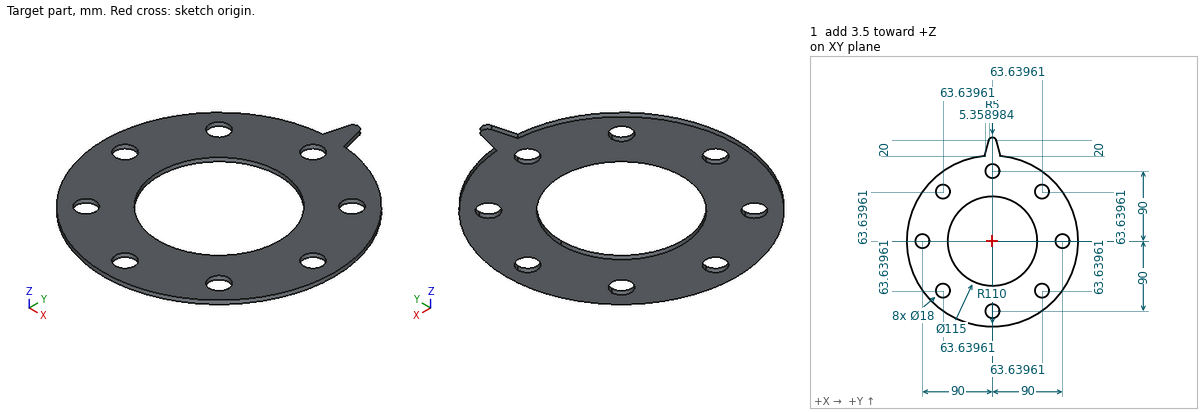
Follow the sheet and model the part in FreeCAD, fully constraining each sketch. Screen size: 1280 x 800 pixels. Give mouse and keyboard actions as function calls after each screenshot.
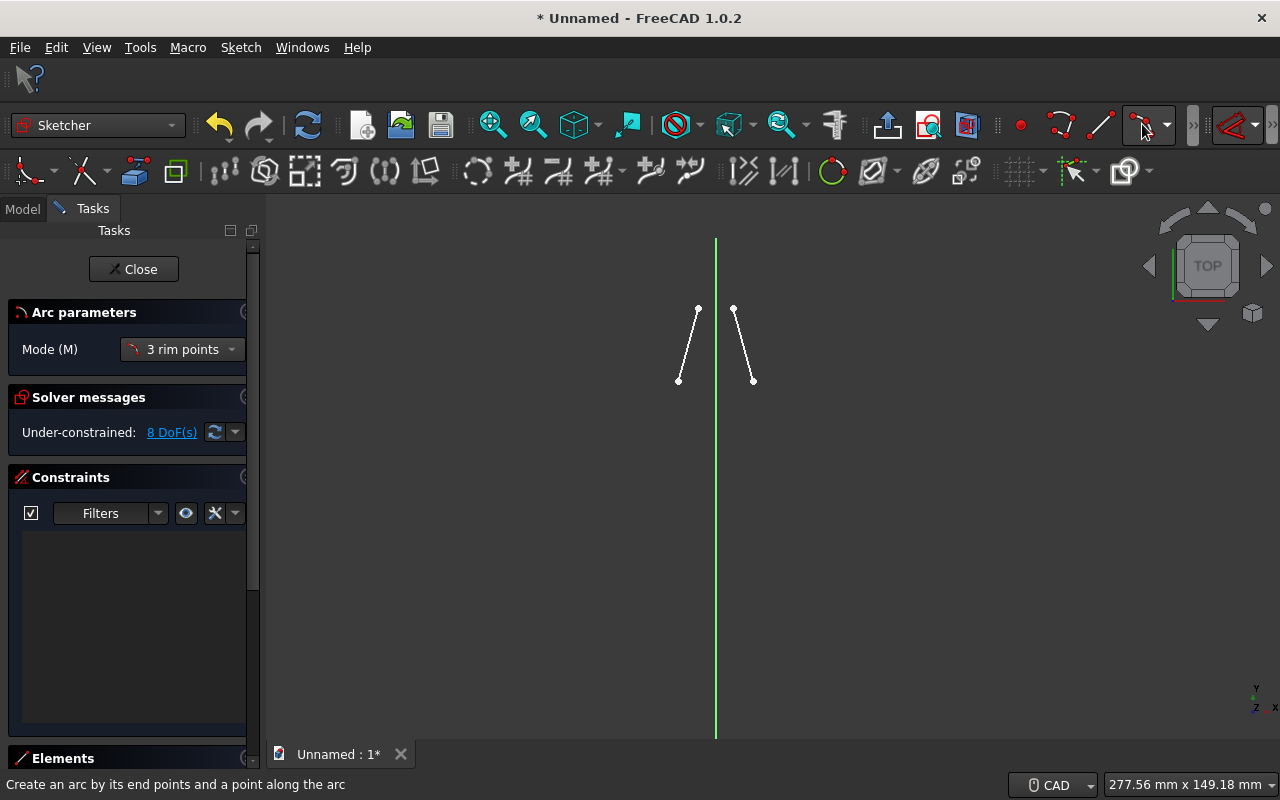
click(678, 381)
click(753, 381)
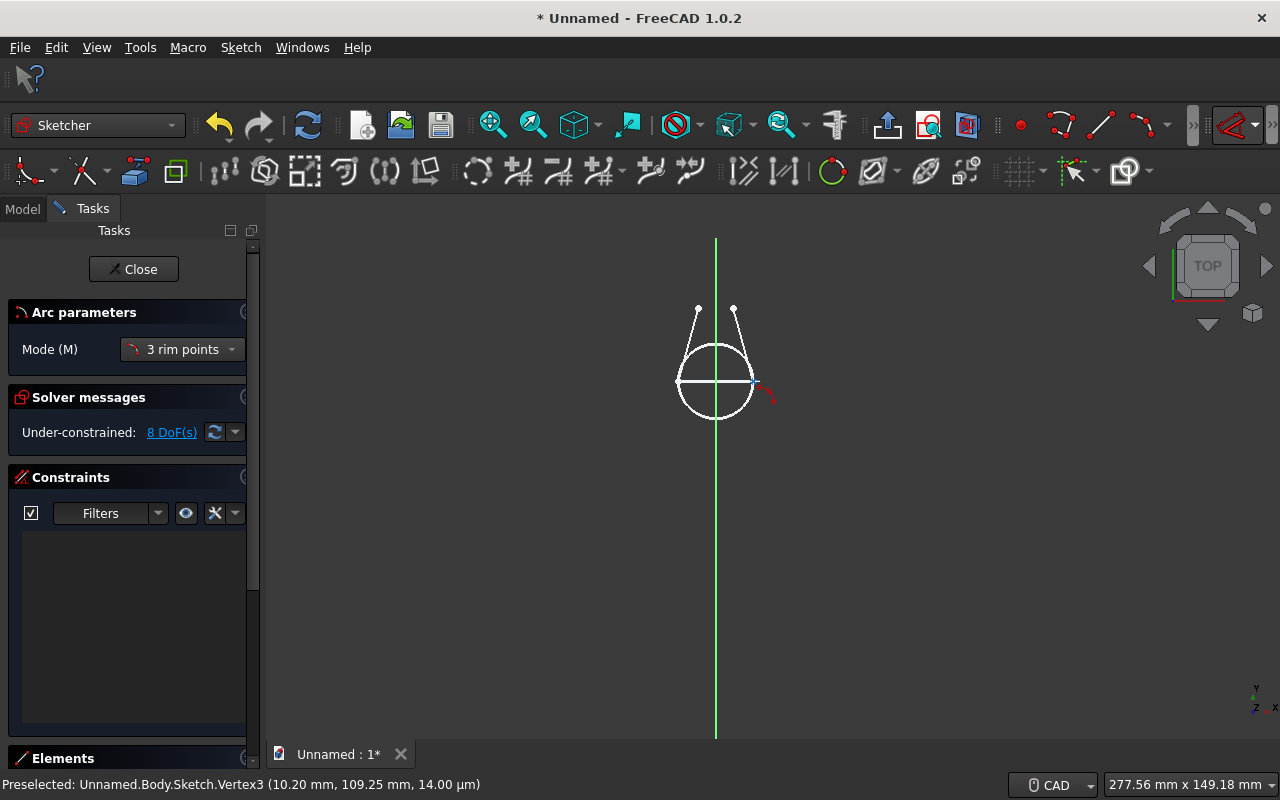
scroll(698, 309, down, 5)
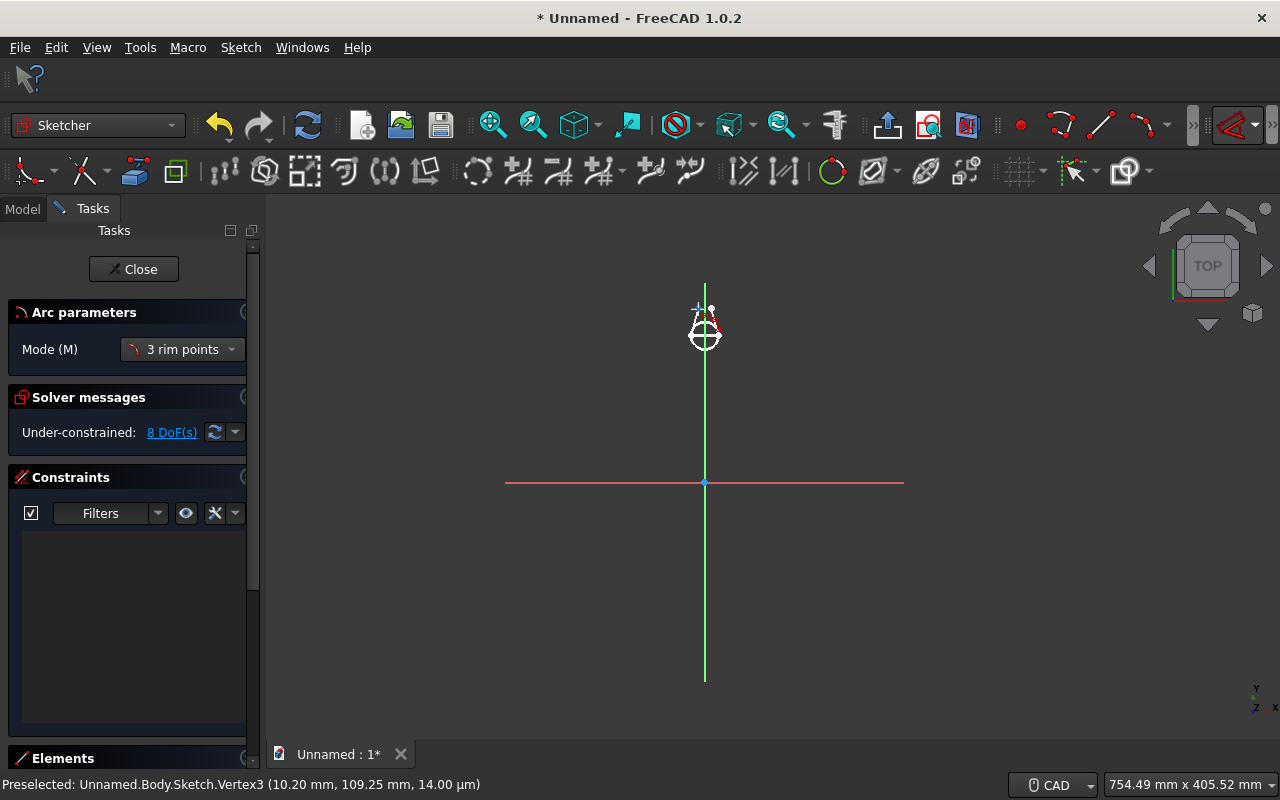
click(620, 604)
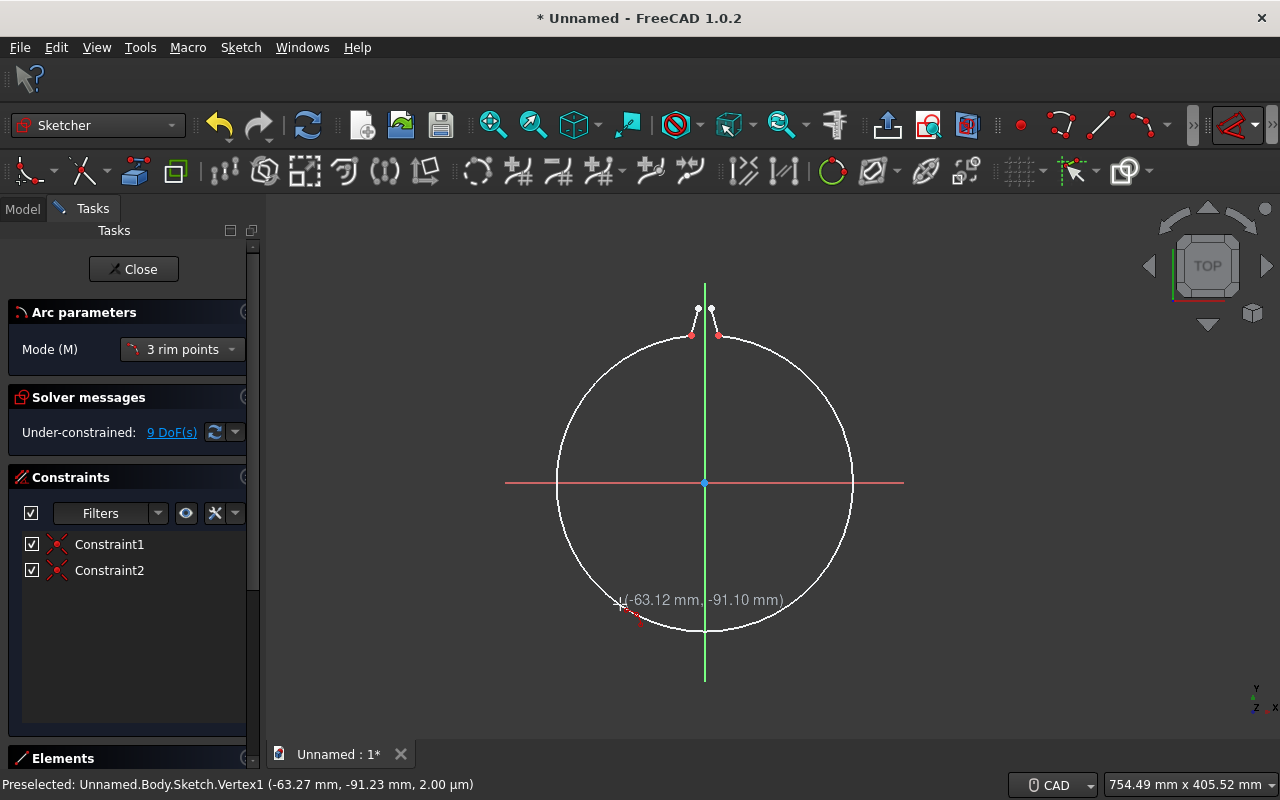
scroll(711, 308, up, 5)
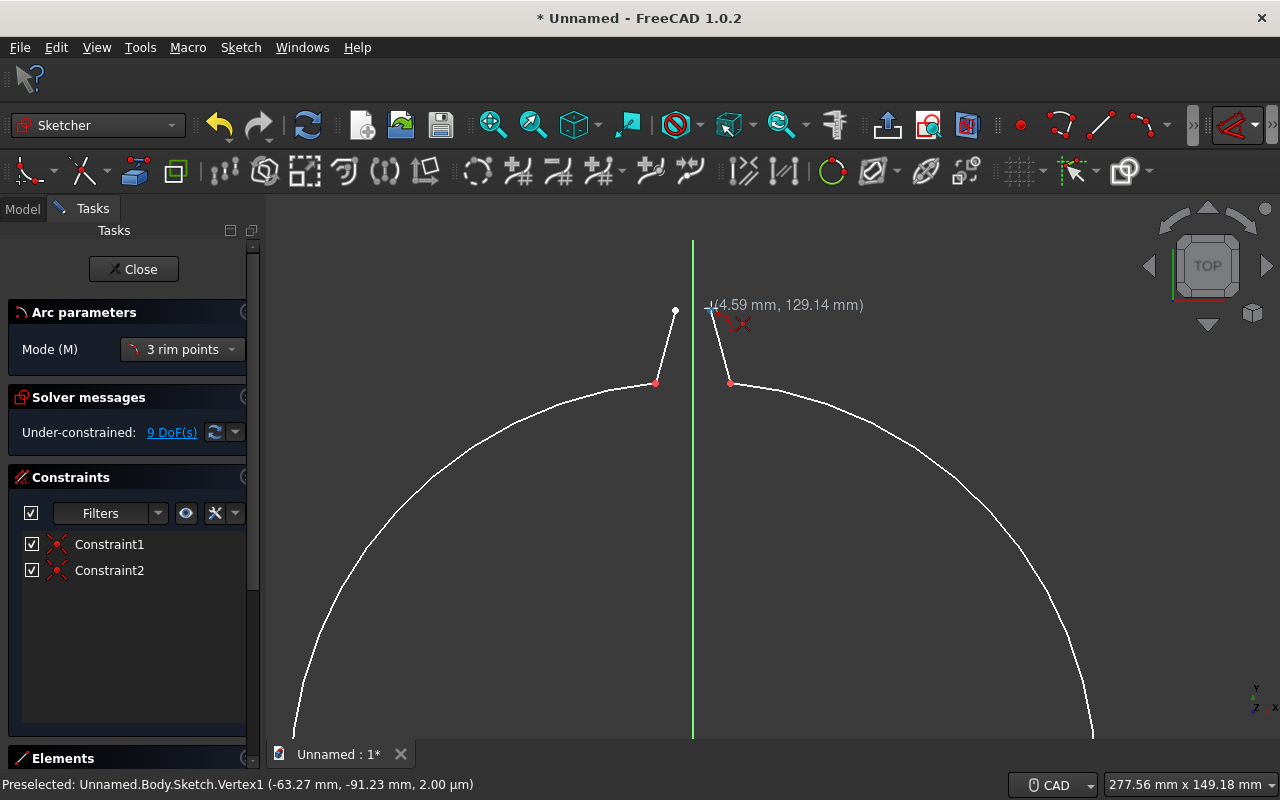
click(711, 310)
click(676, 310)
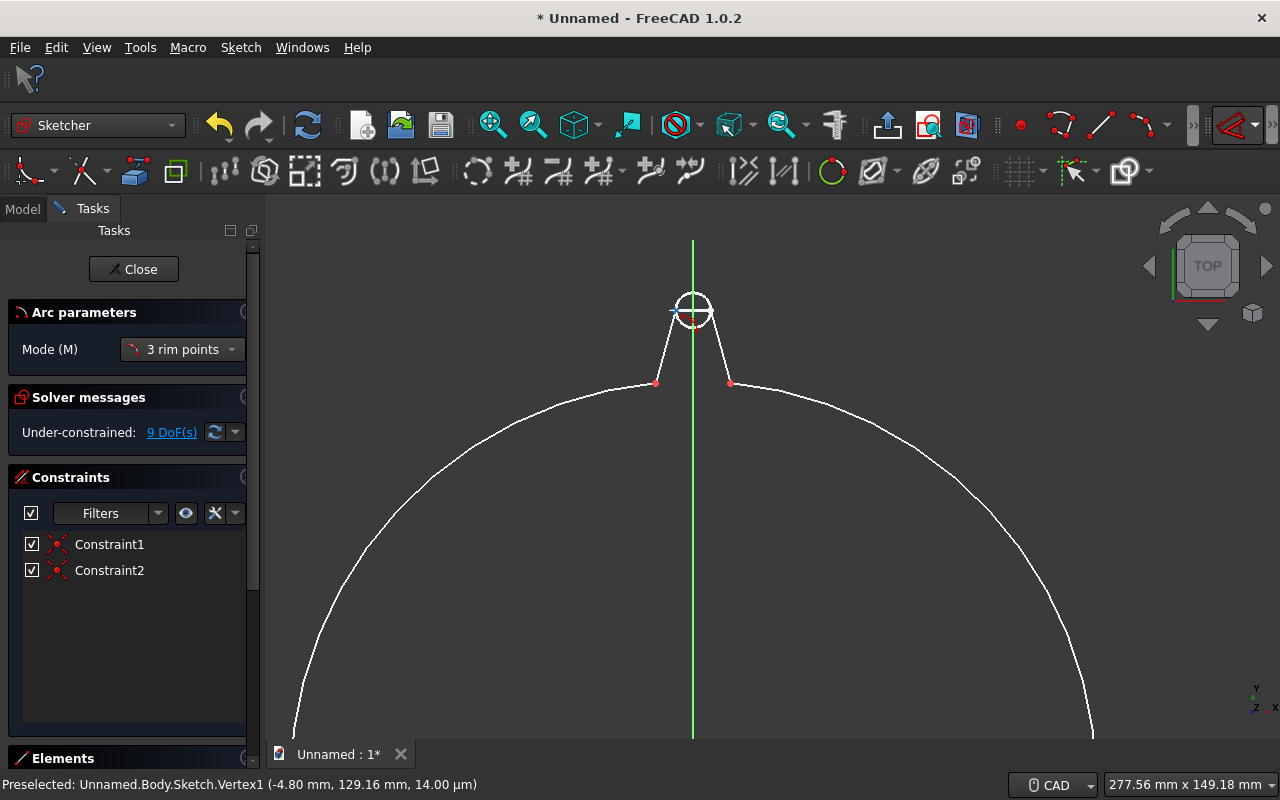
scroll(703, 298, up, 3)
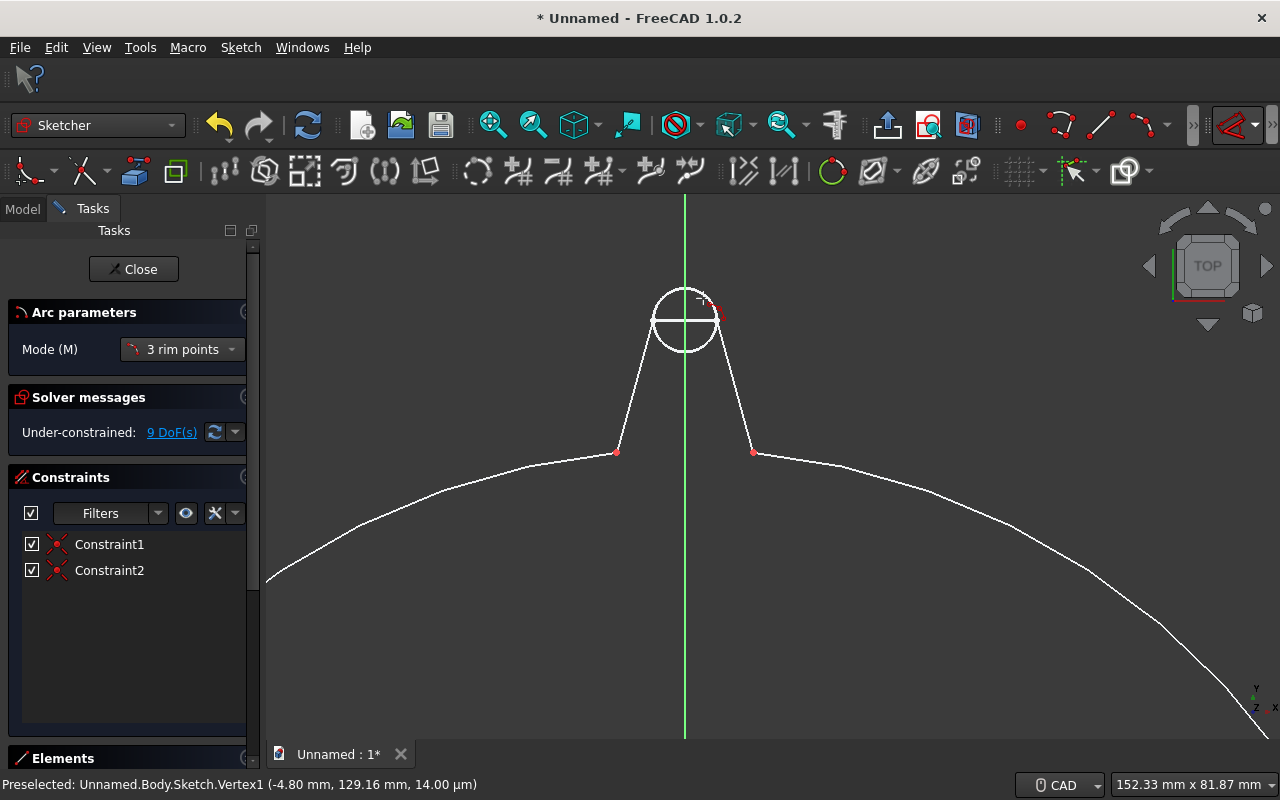
click(702, 298)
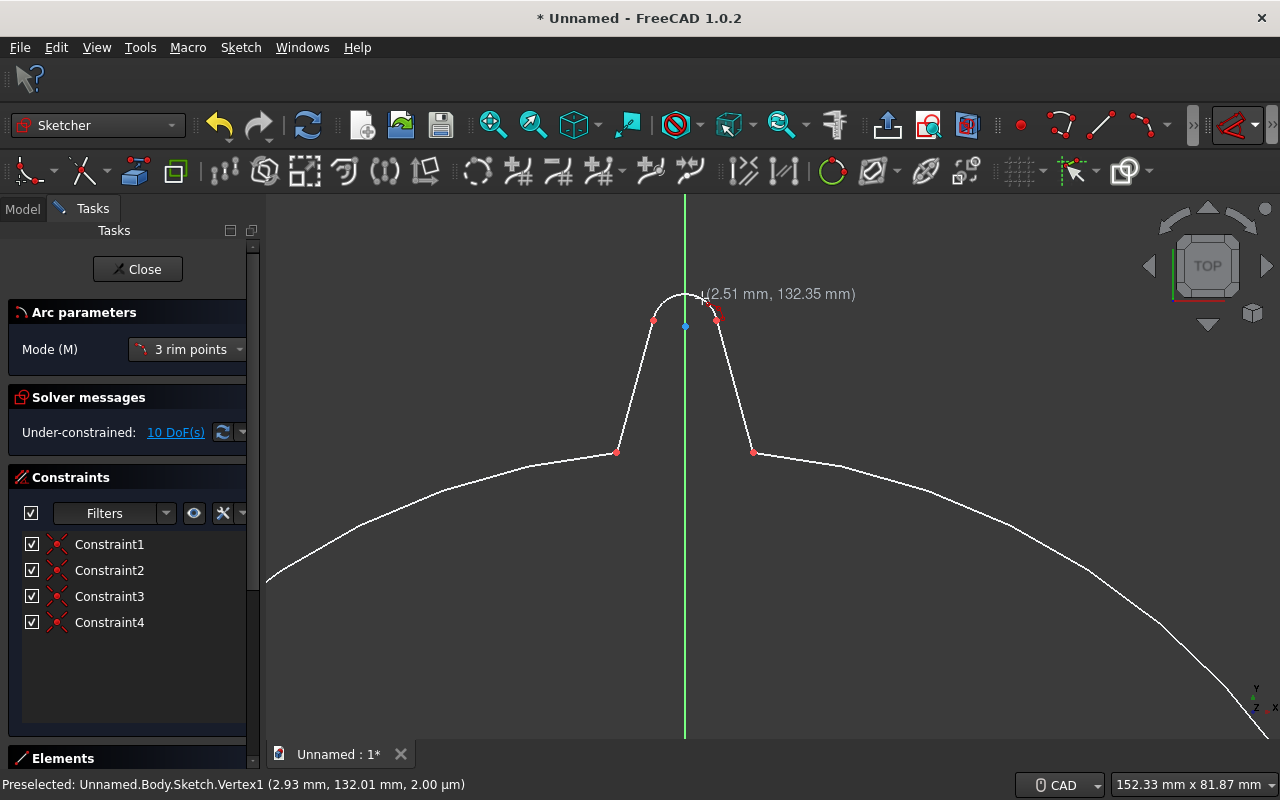
key(g)
key(c)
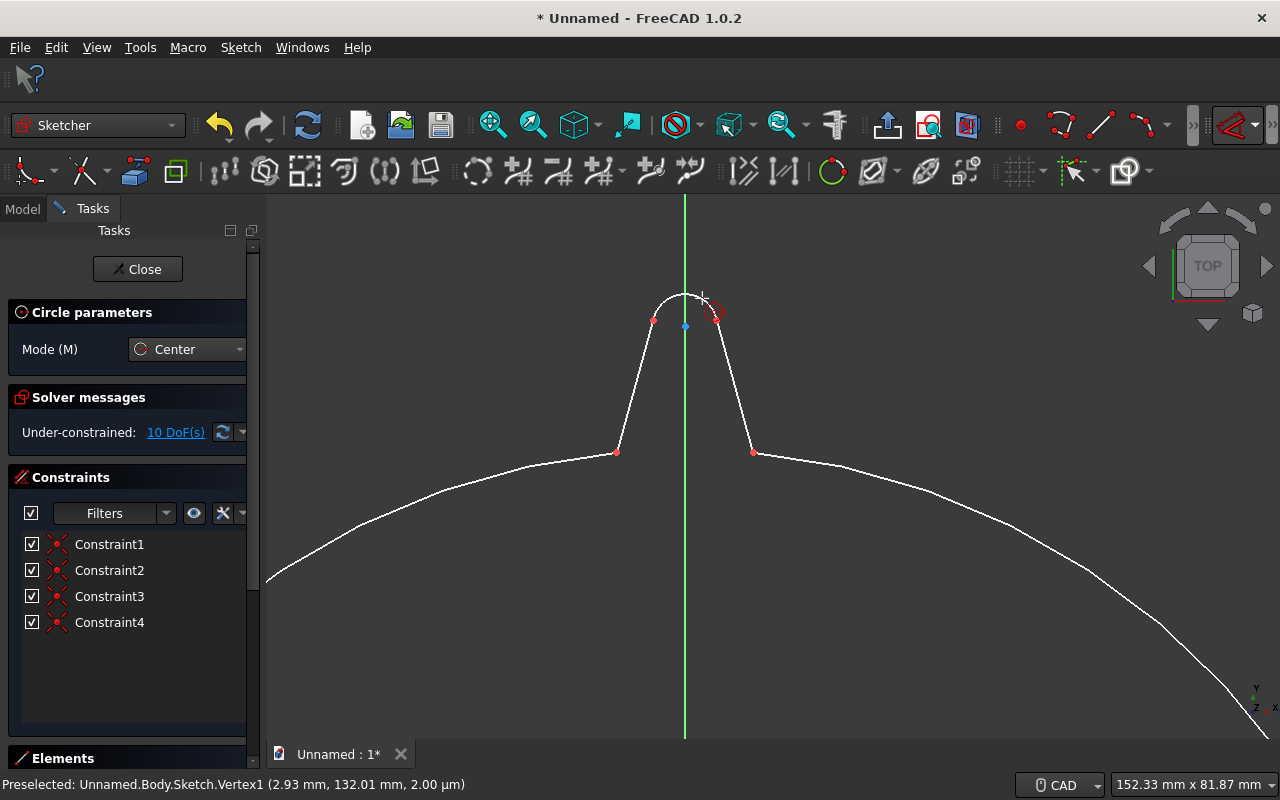
scroll(709, 306, down, 8)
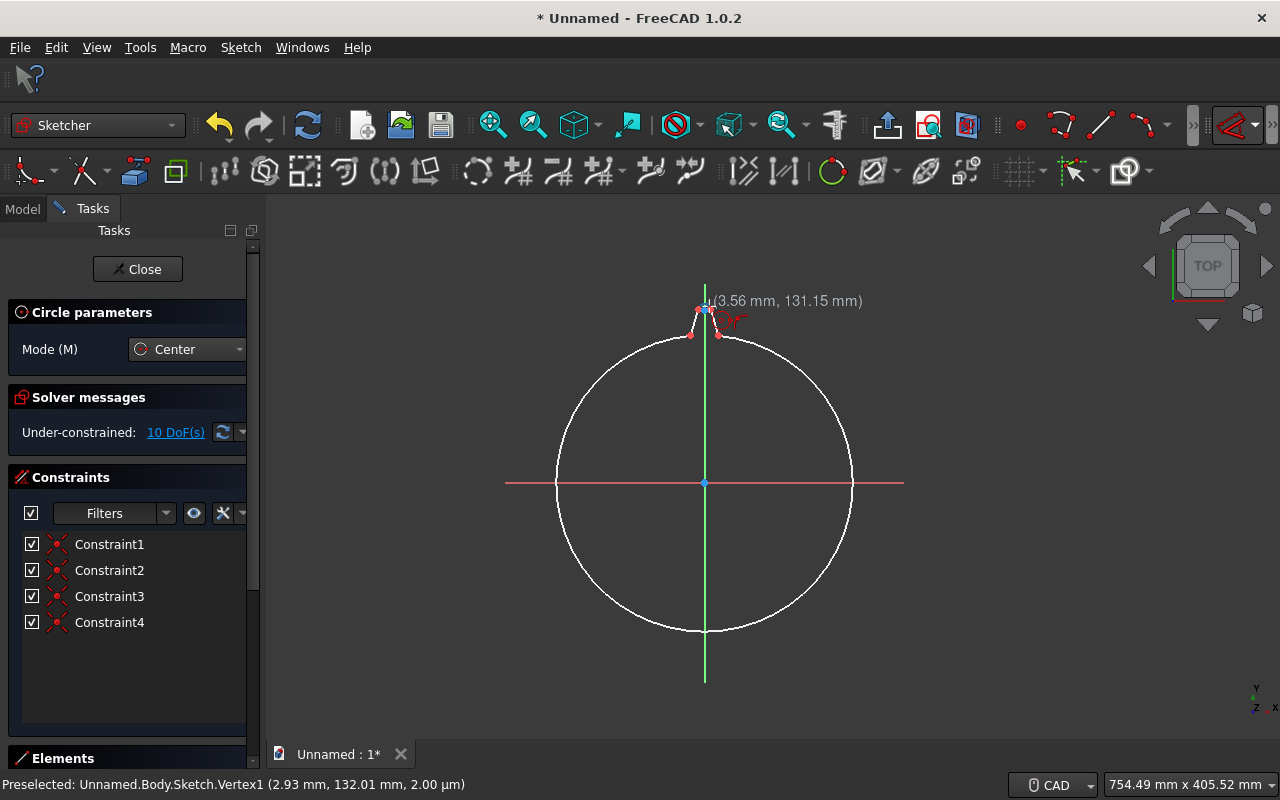
scroll(619, 568, up, 4)